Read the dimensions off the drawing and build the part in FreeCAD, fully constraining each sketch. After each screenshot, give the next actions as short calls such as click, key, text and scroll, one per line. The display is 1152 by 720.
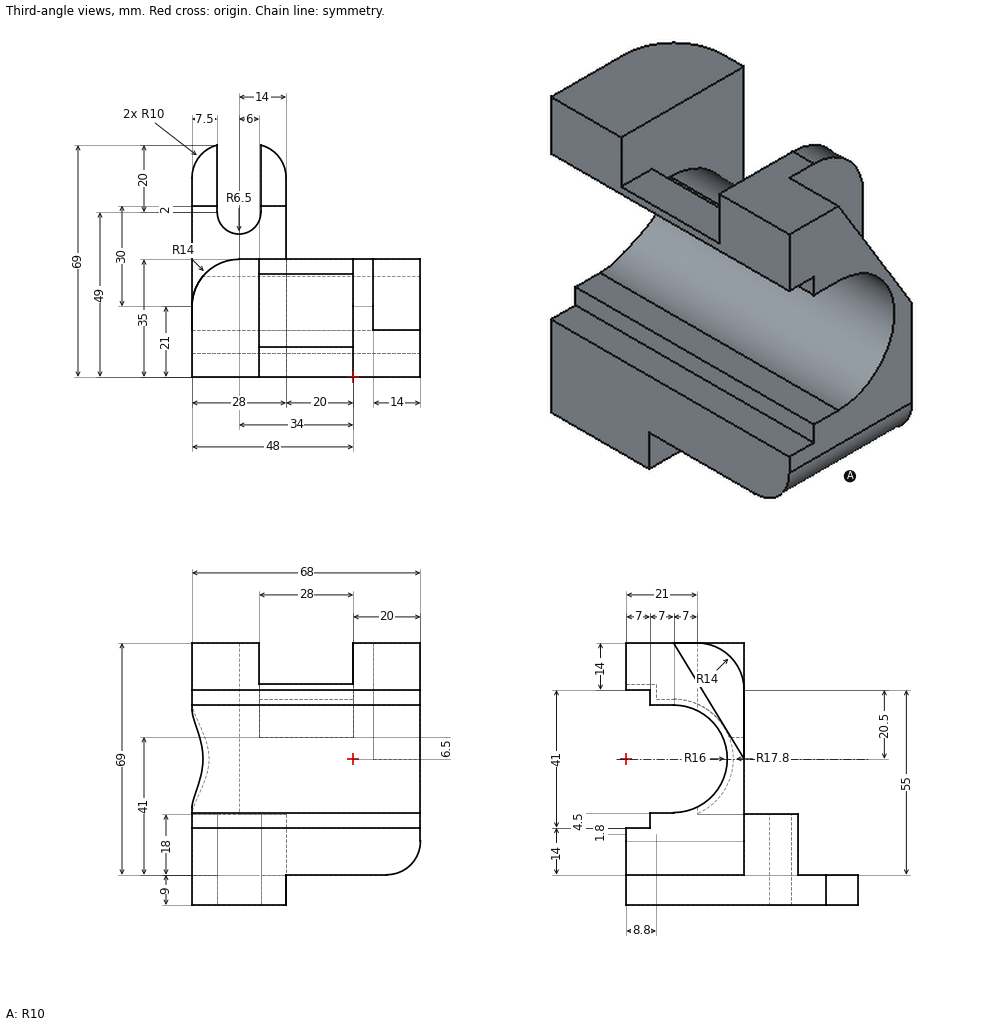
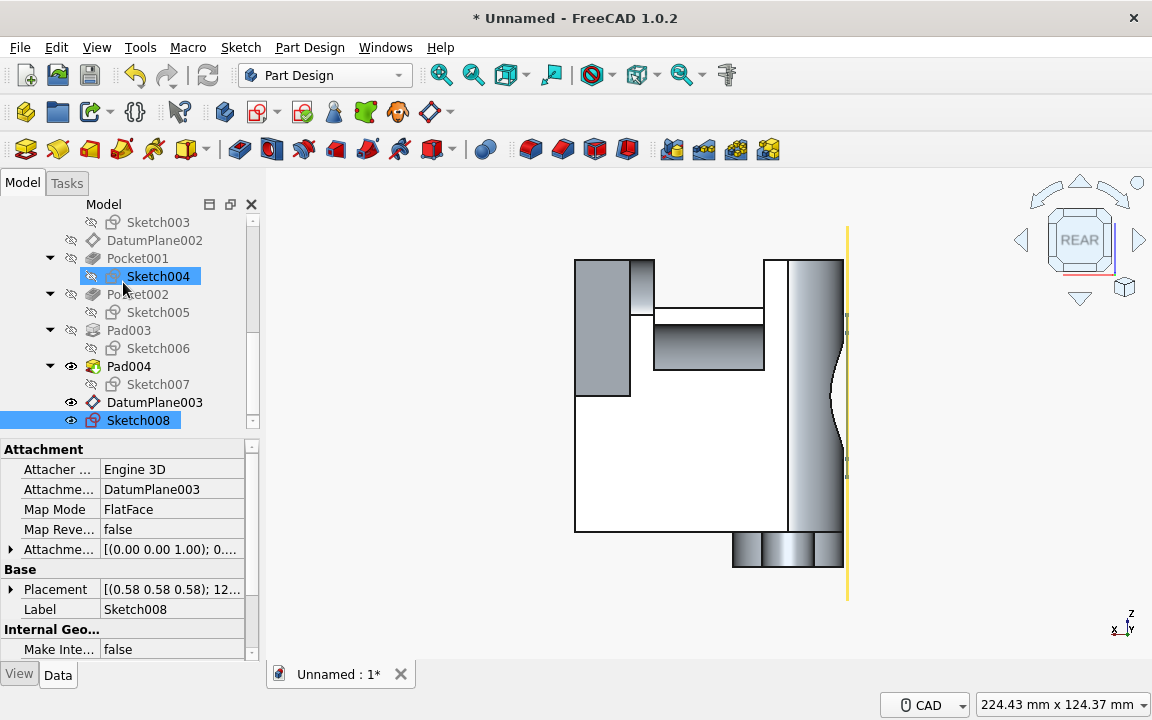
click(240, 150)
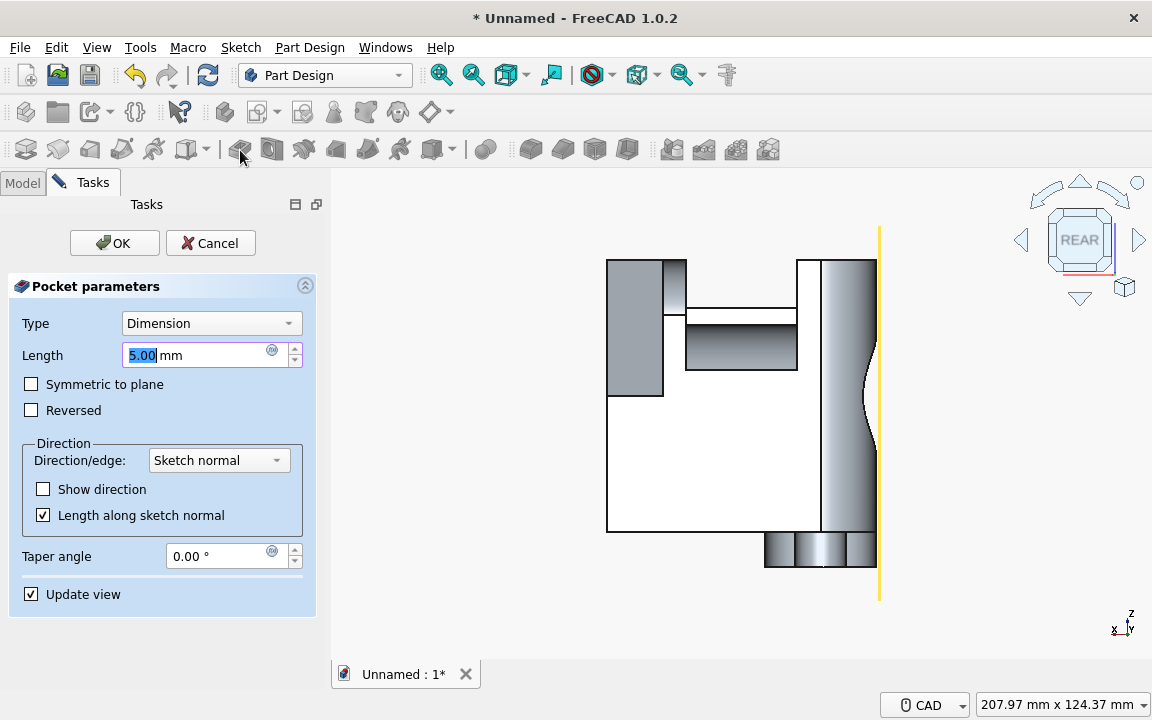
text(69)
key(Tab)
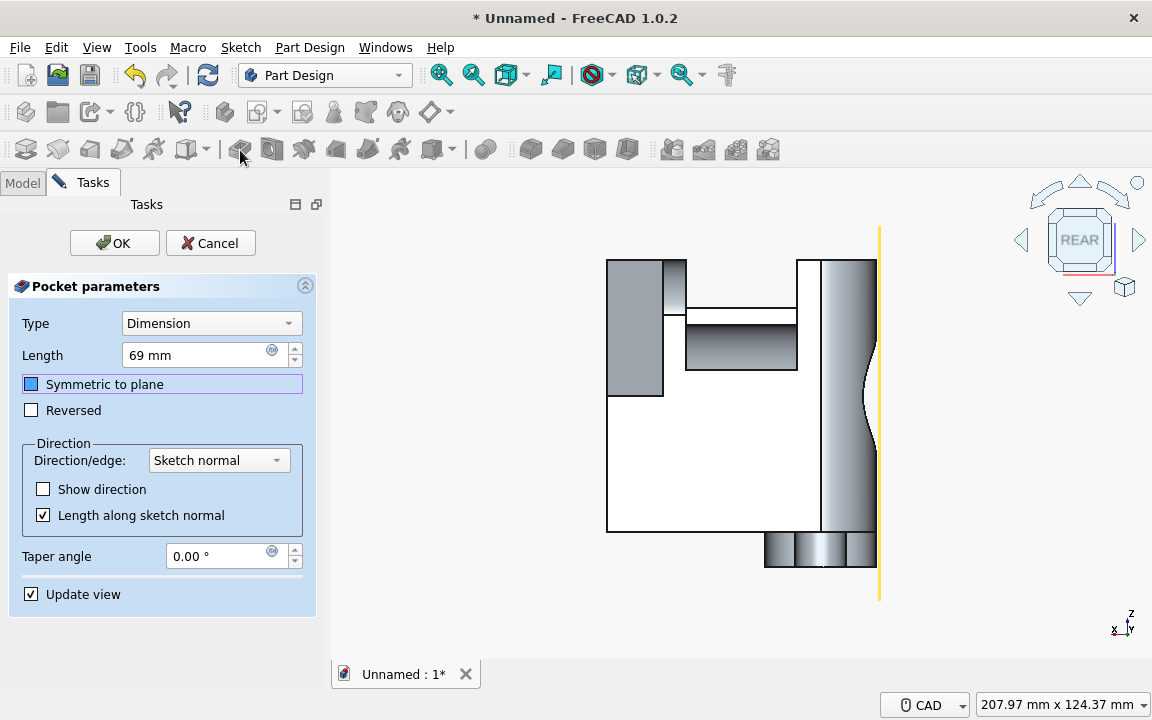
click(30, 410)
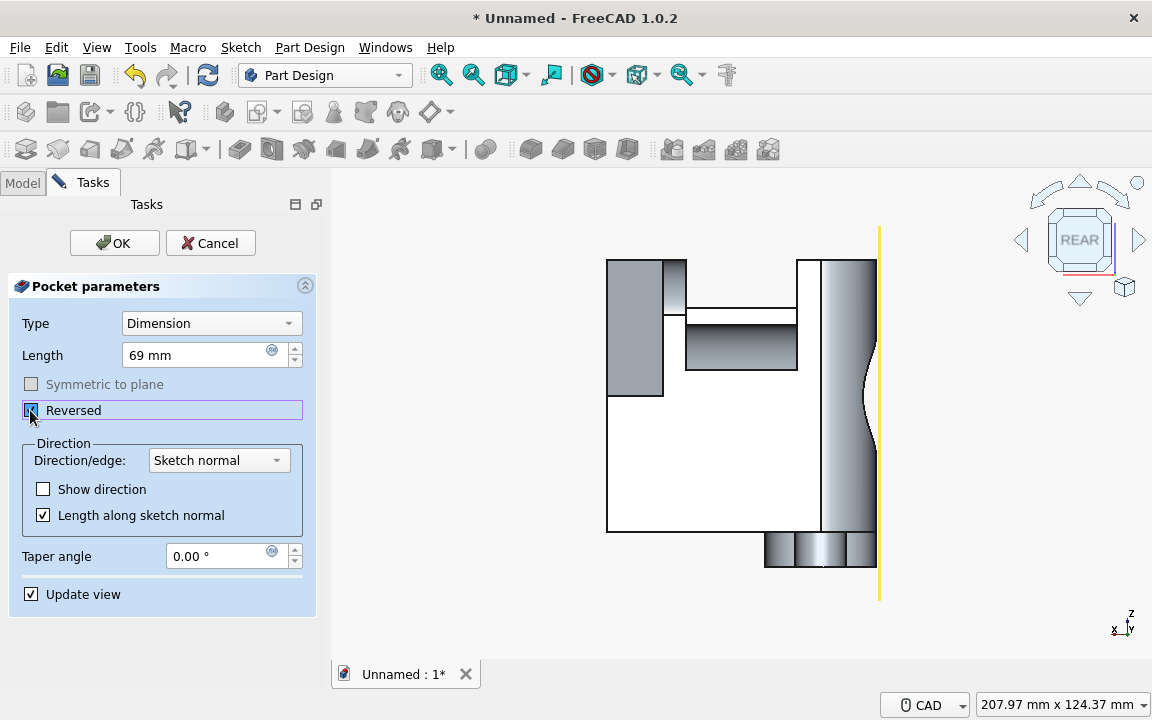
click(115, 243)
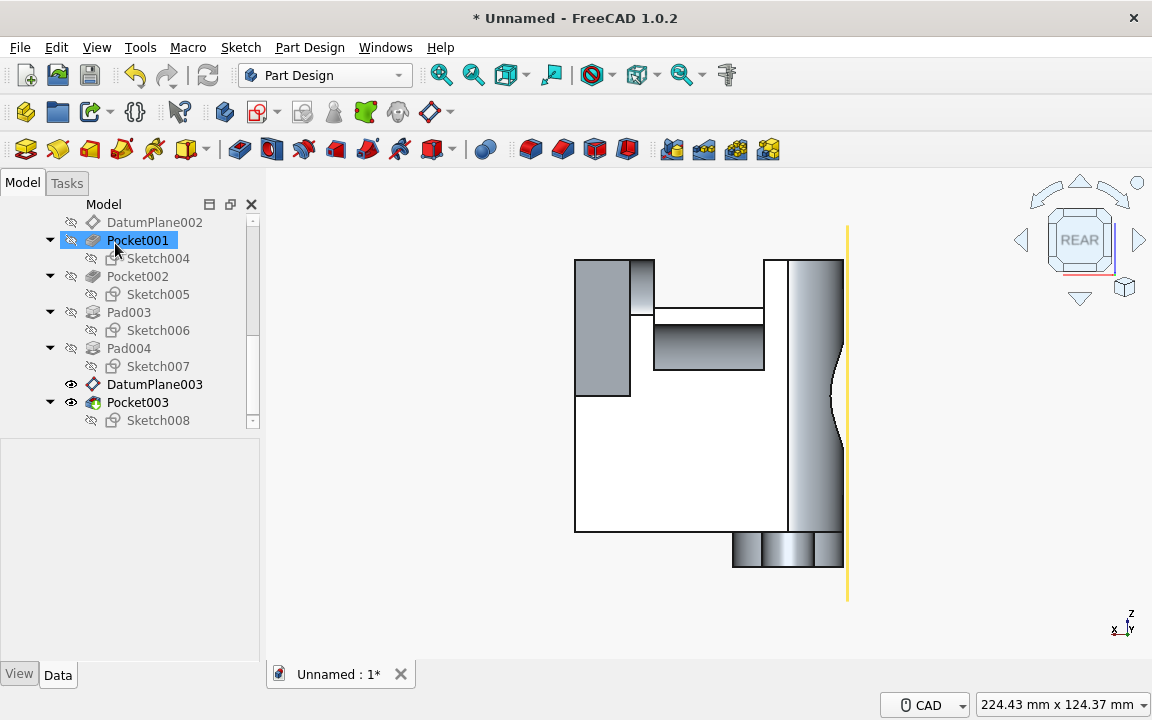
click(116, 384)
key(space)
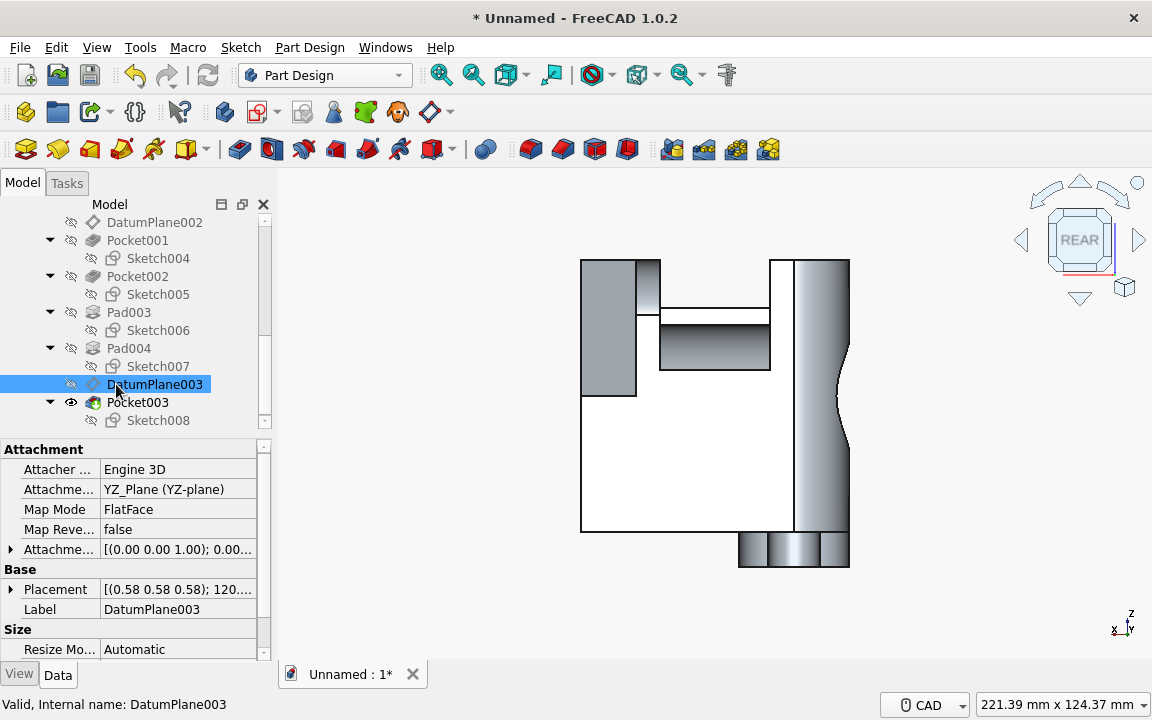
scroll(140, 326, down, 3)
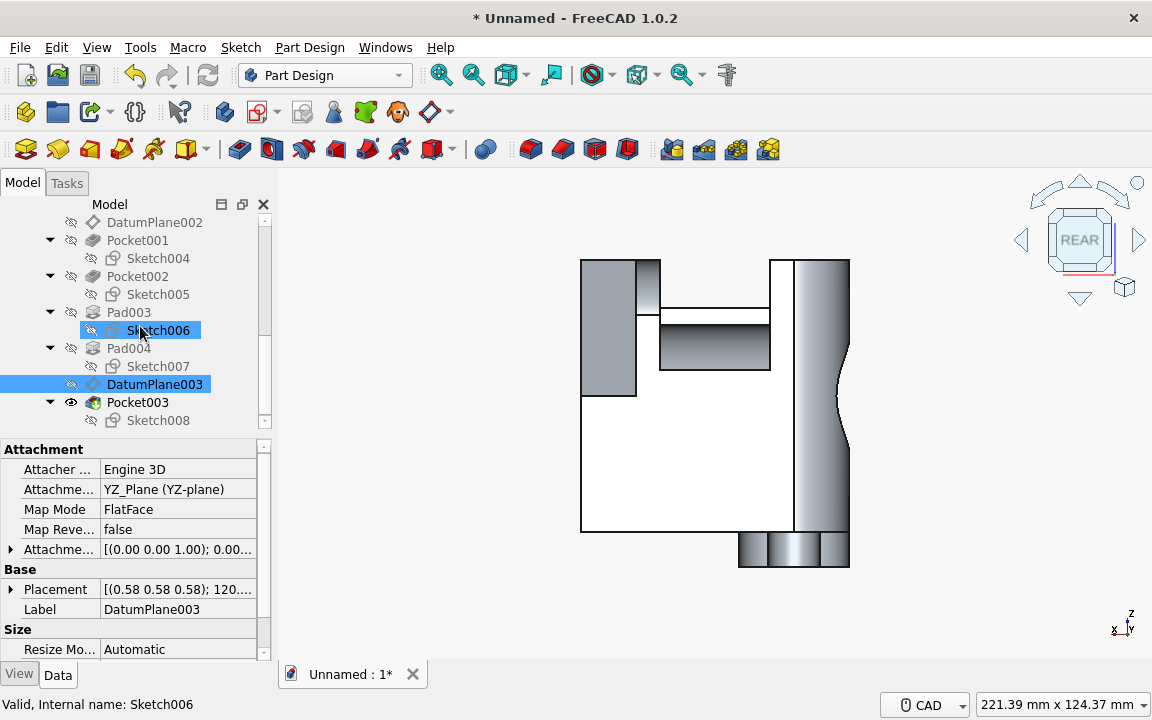
scroll(140, 326, up, 15)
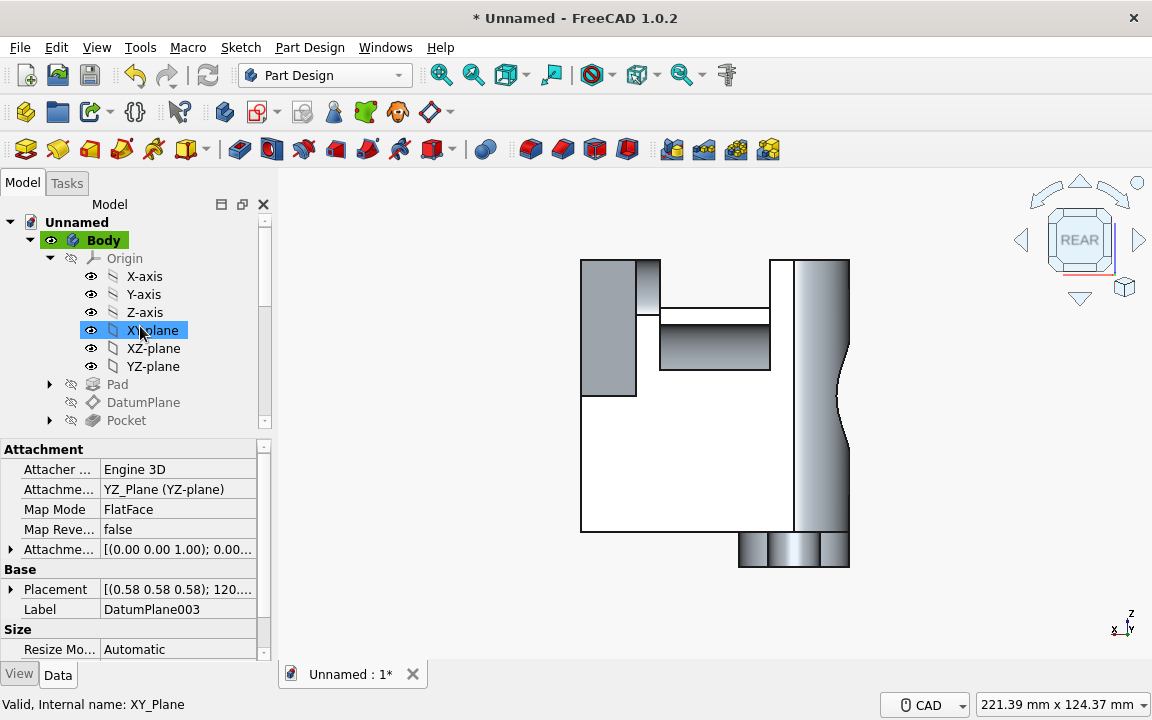
click(136, 330)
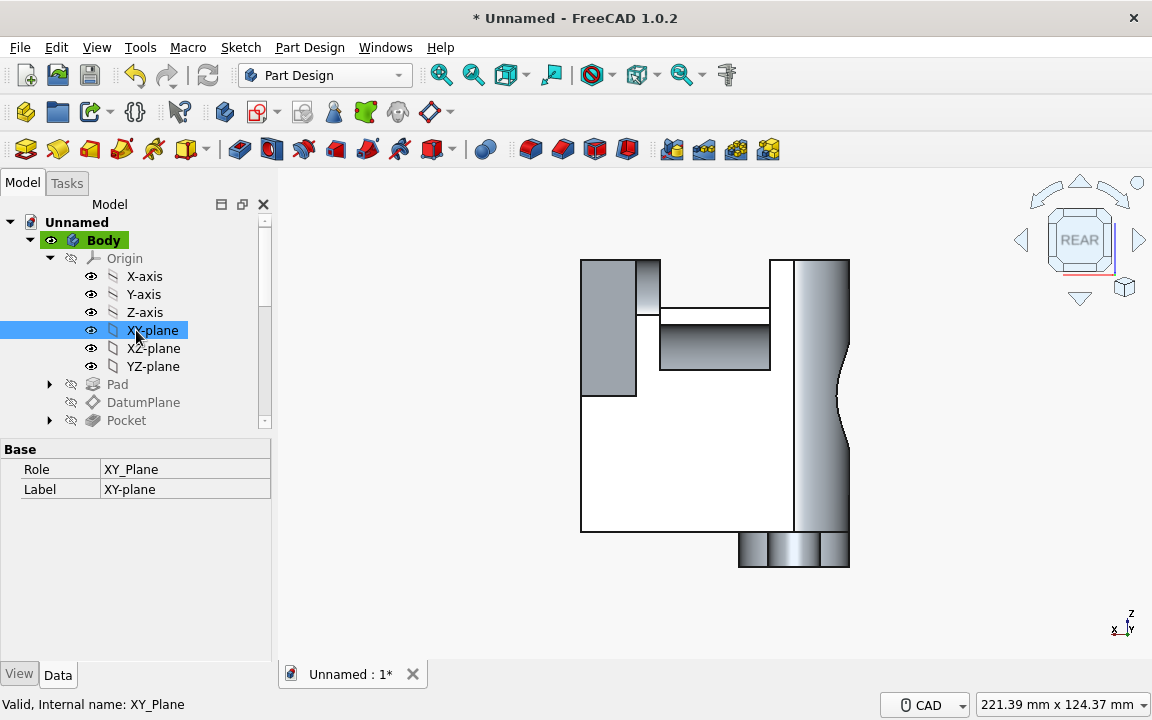
click(430, 112)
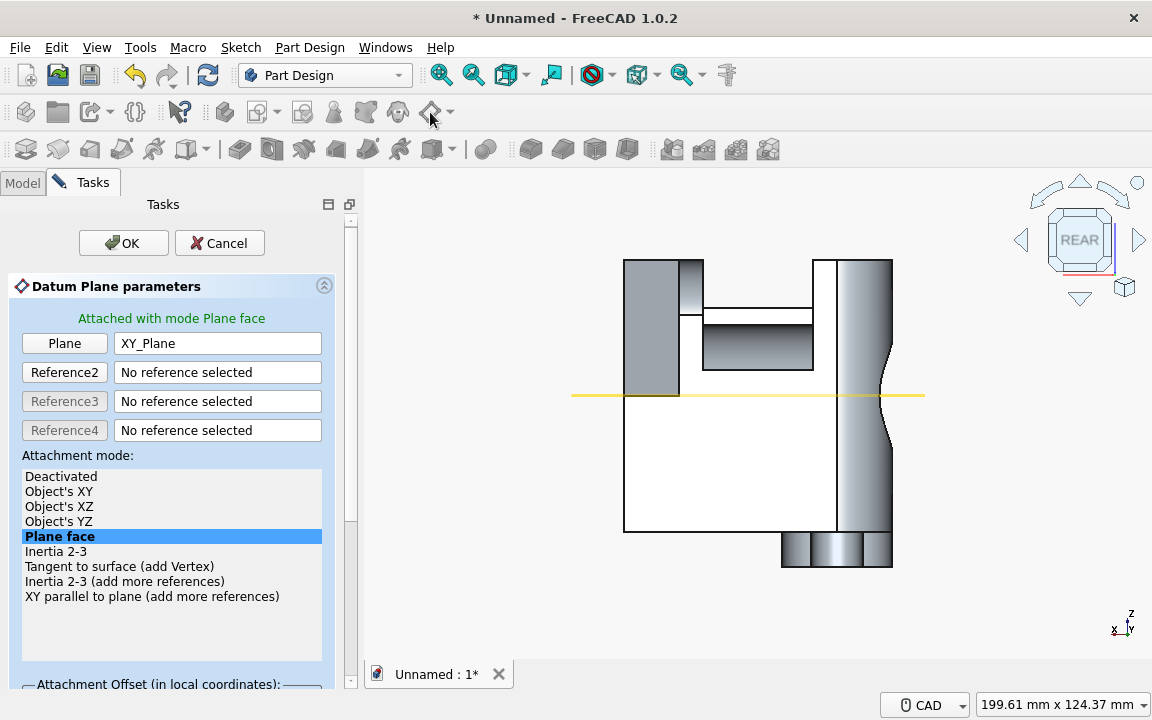
scroll(351, 451, down, 3)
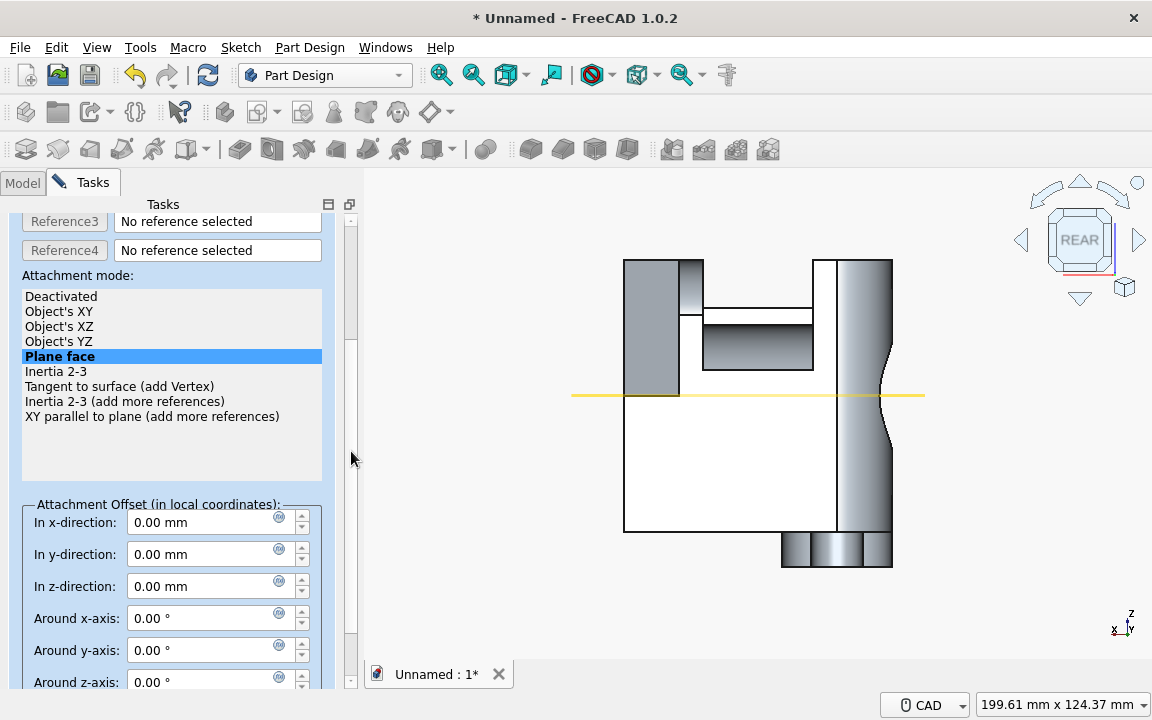
triple_click(210, 586)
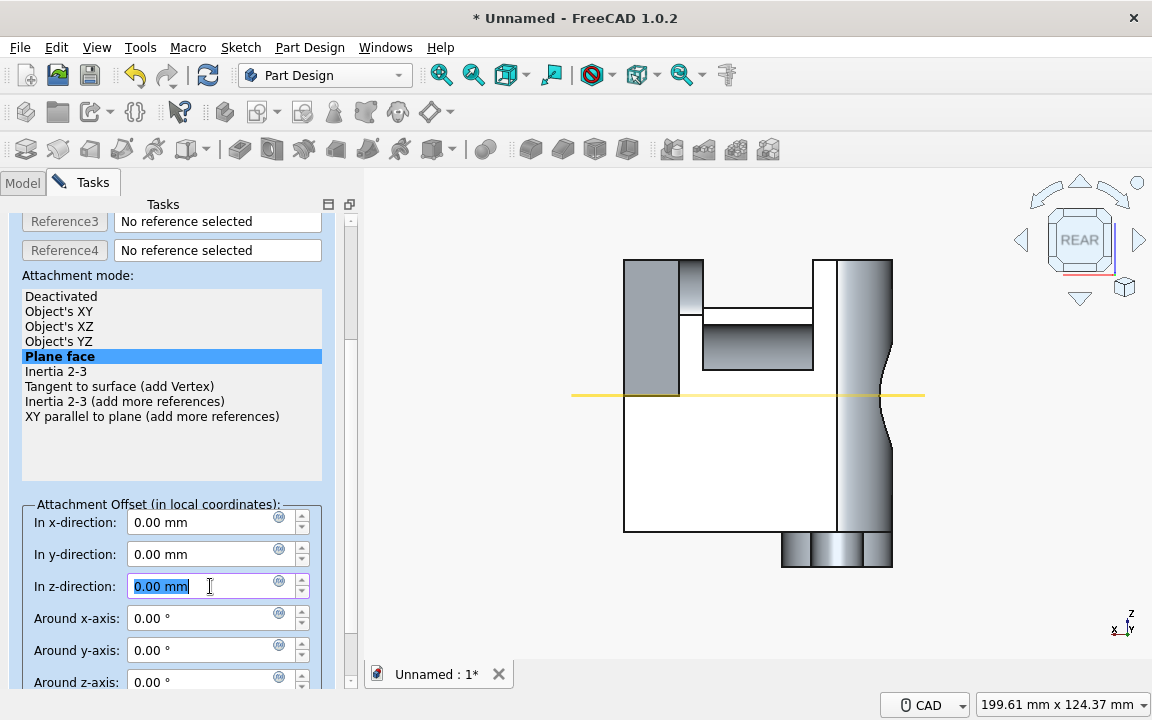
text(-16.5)
key(Tab)